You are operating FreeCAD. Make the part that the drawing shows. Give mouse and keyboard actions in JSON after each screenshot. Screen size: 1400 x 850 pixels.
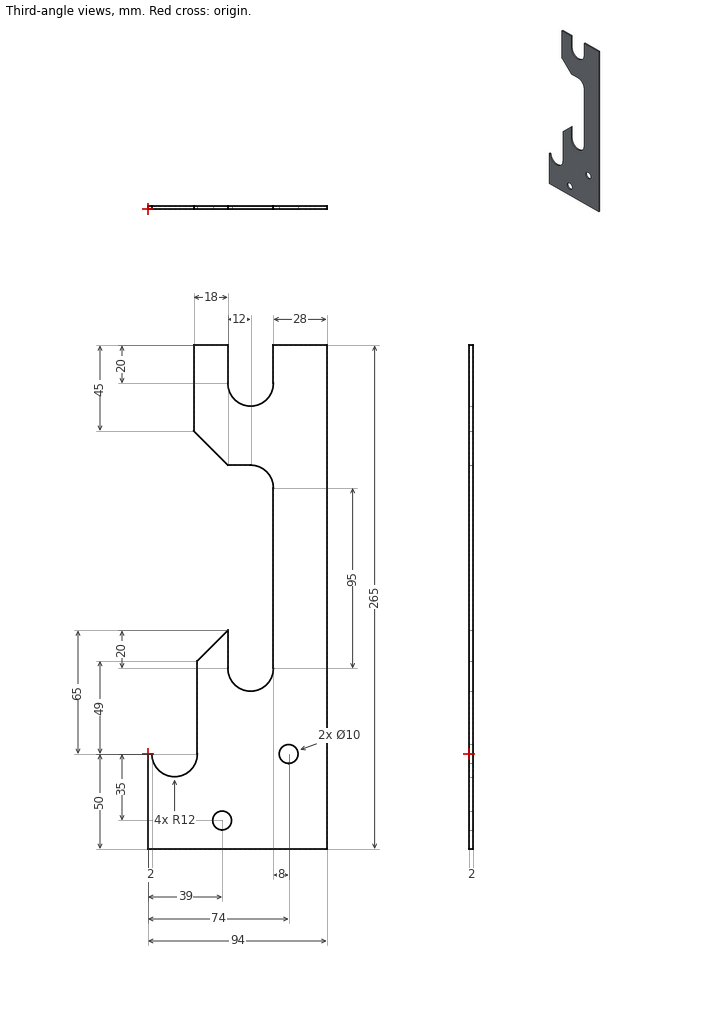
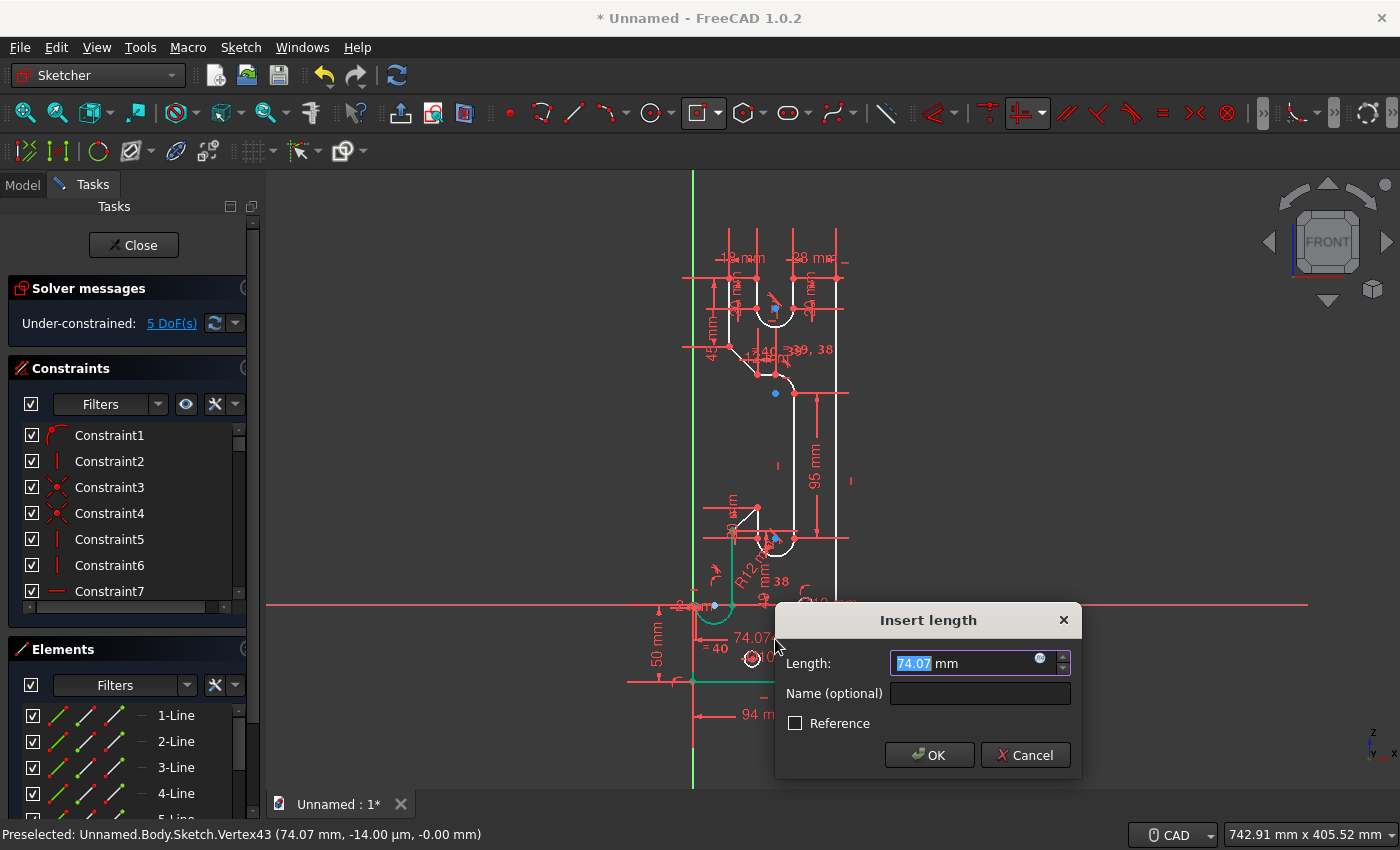
{"action": "type", "text": "74"}
{"action": "key", "text": "Return"}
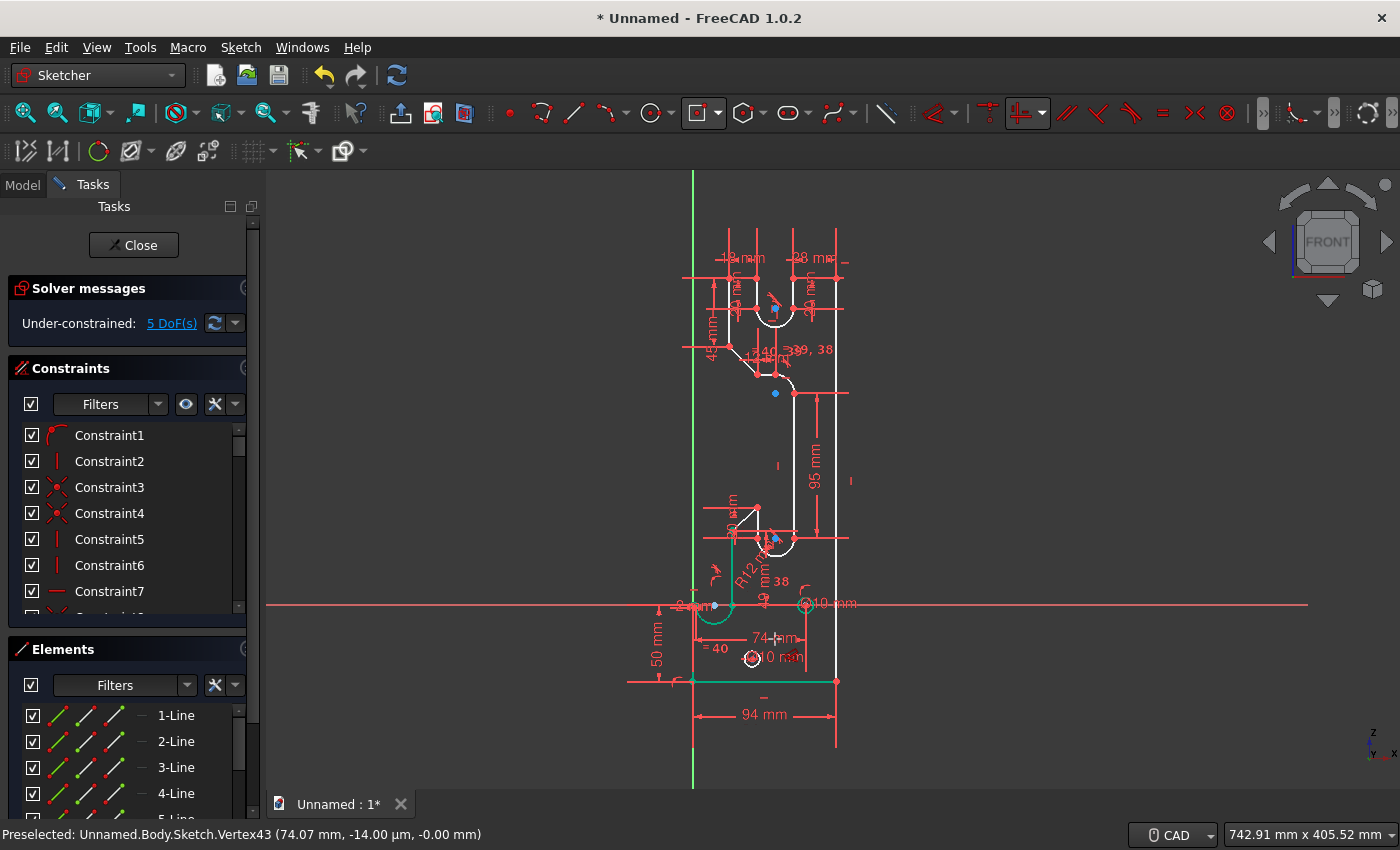
{"action": "left_click", "coordinate": [752, 659]}
{"action": "left_click", "coordinate": [722, 741]}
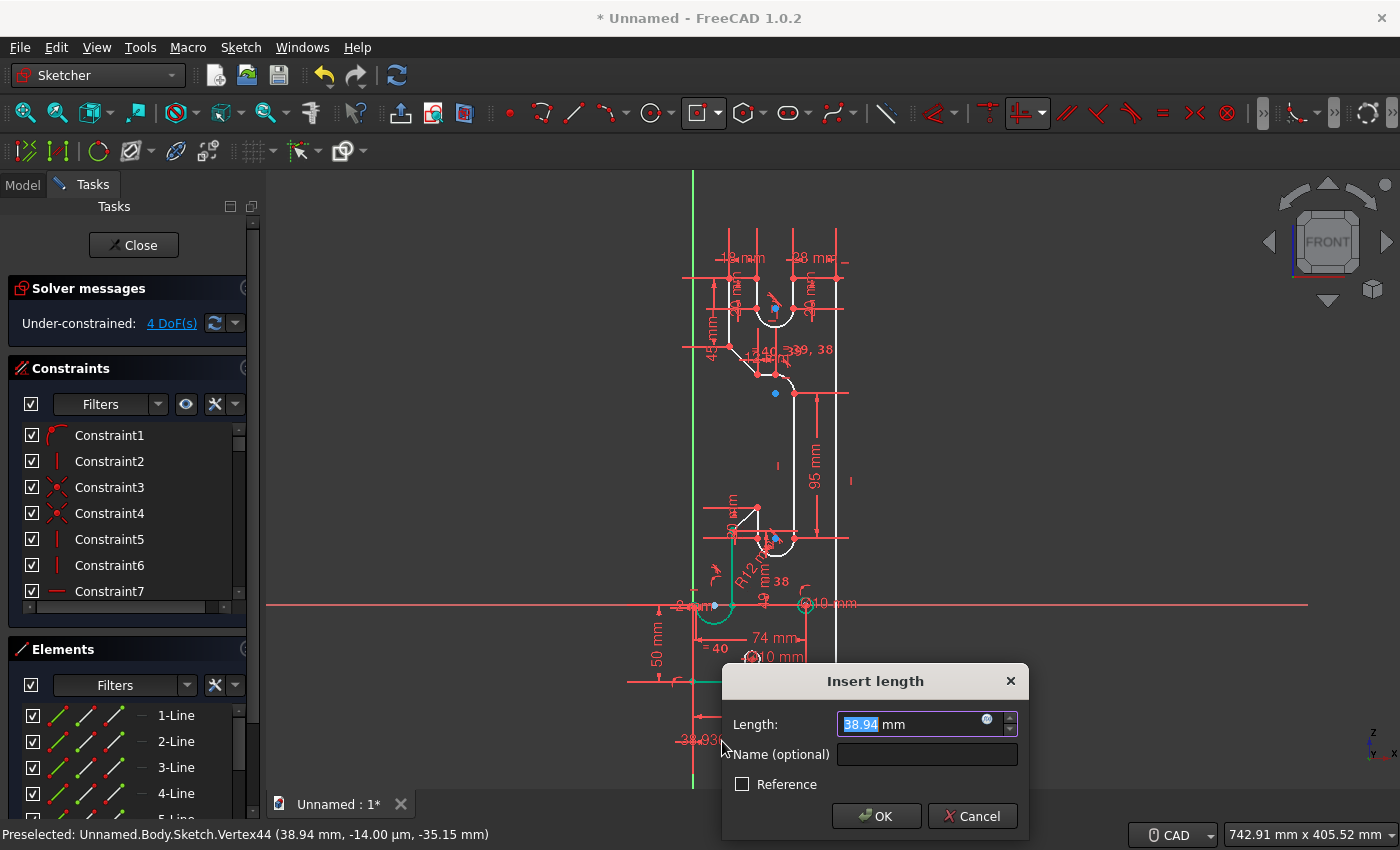
{"action": "type", "text": "39"}
{"action": "key", "text": "Return"}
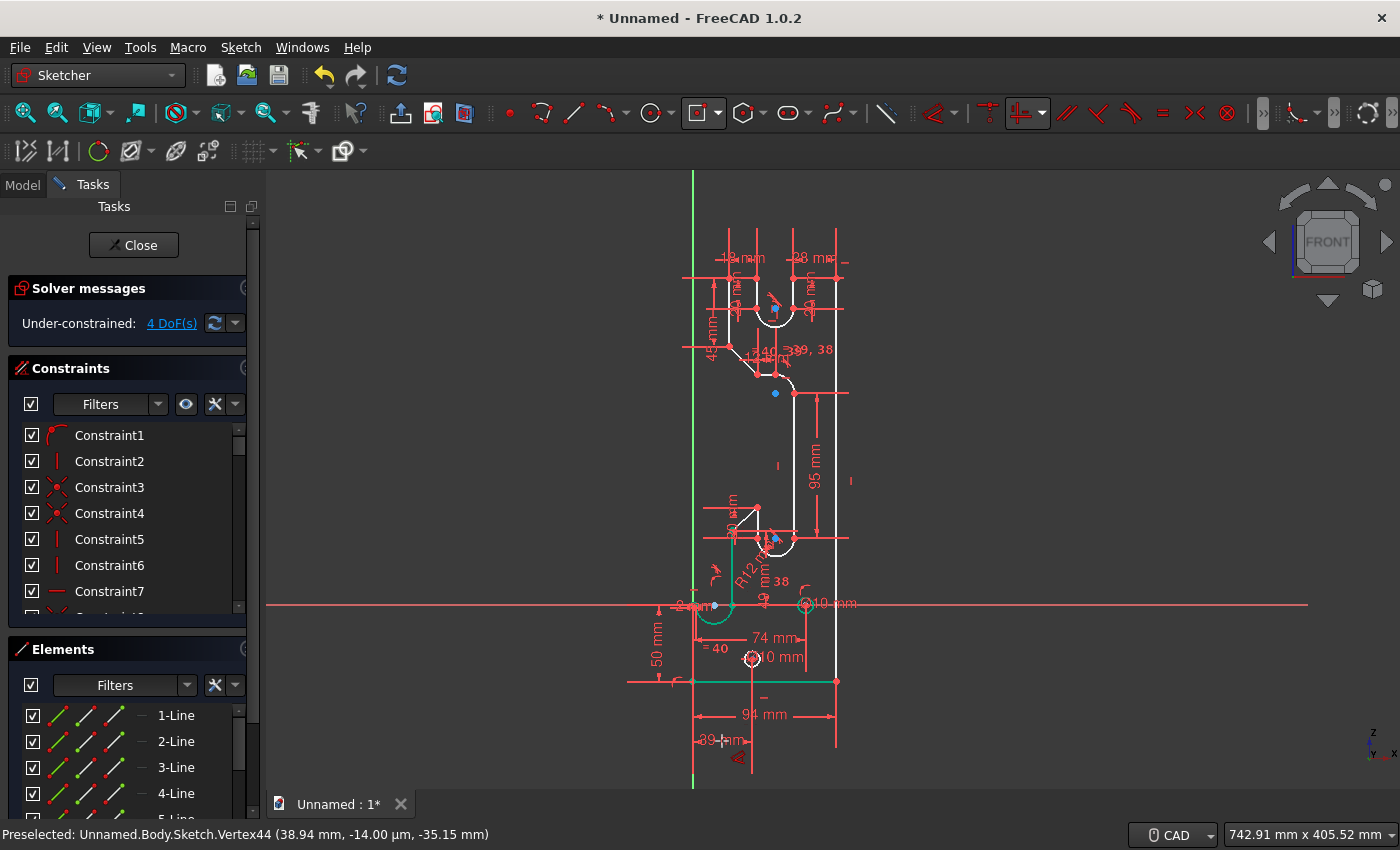
{"action": "left_click", "coordinate": [752, 659]}
{"action": "left_click", "coordinate": [611, 620]}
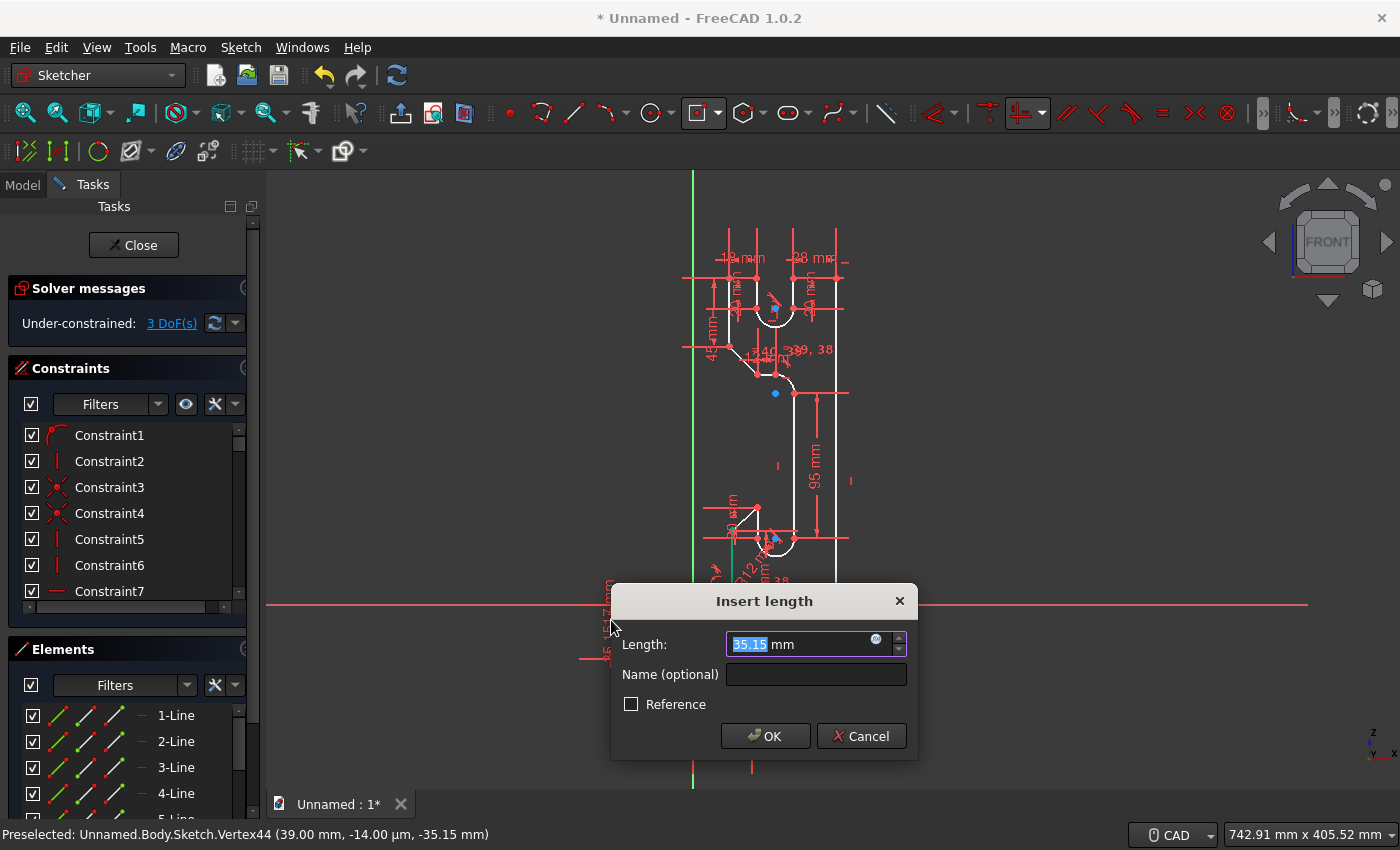
{"action": "type", "text": "35"}
{"action": "key", "text": "Return"}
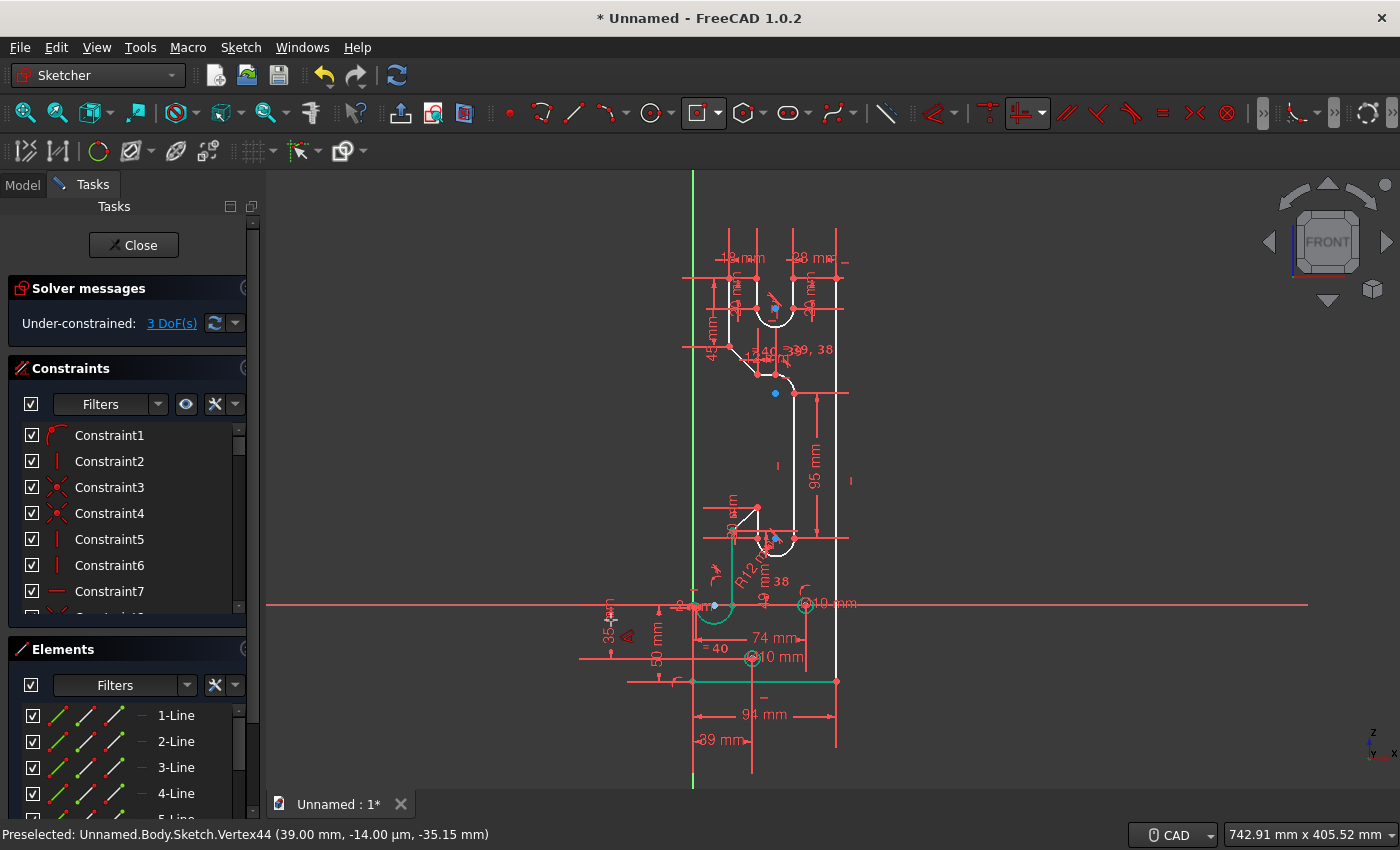
{"action": "scroll", "coordinate": [794, 538], "scroll_direction": "up", "scroll_amount": 6}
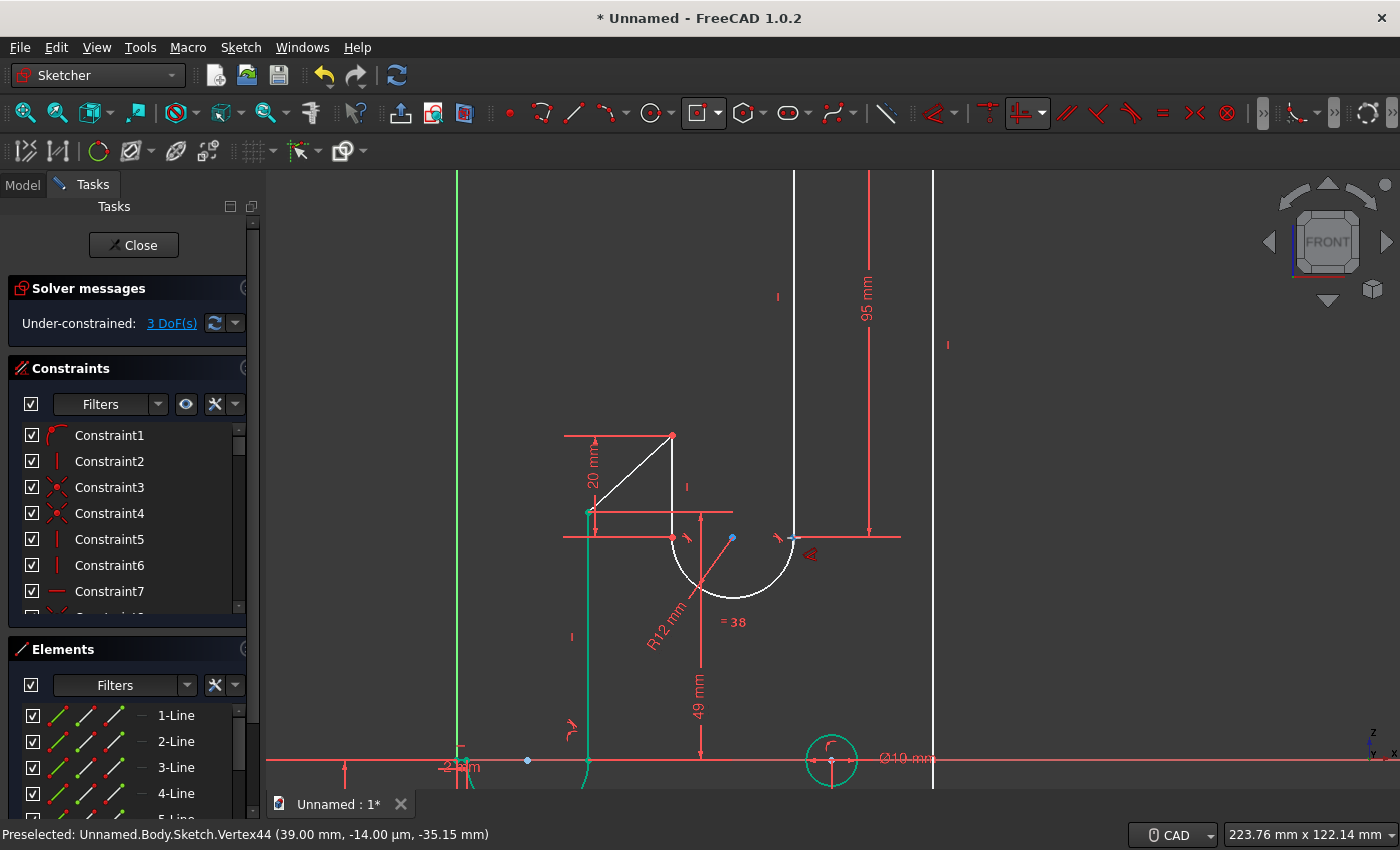
{"action": "left_click", "coordinate": [794, 537]}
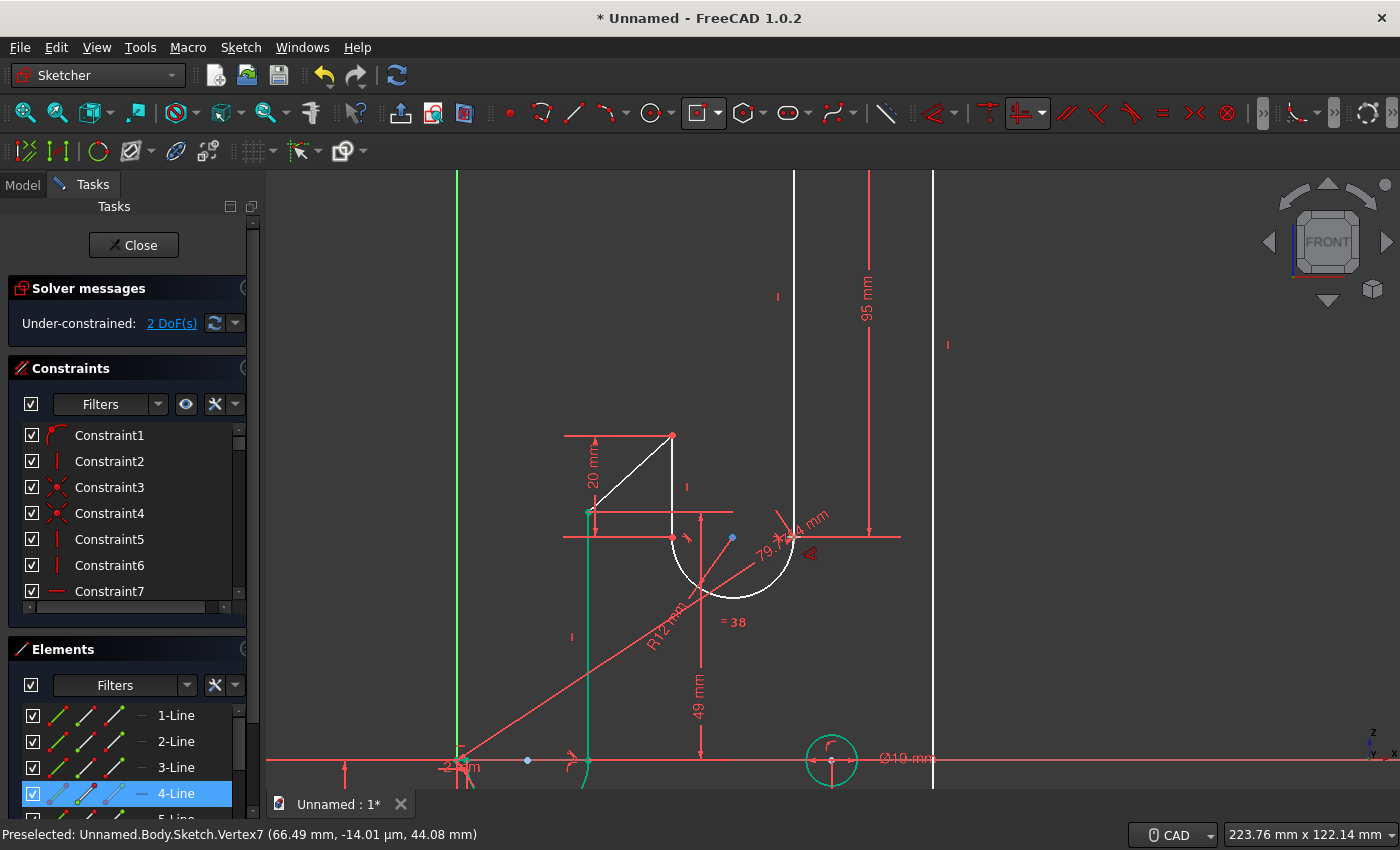
{"action": "left_click", "coordinate": [832, 760]}
{"action": "left_click", "coordinate": [813, 503]}